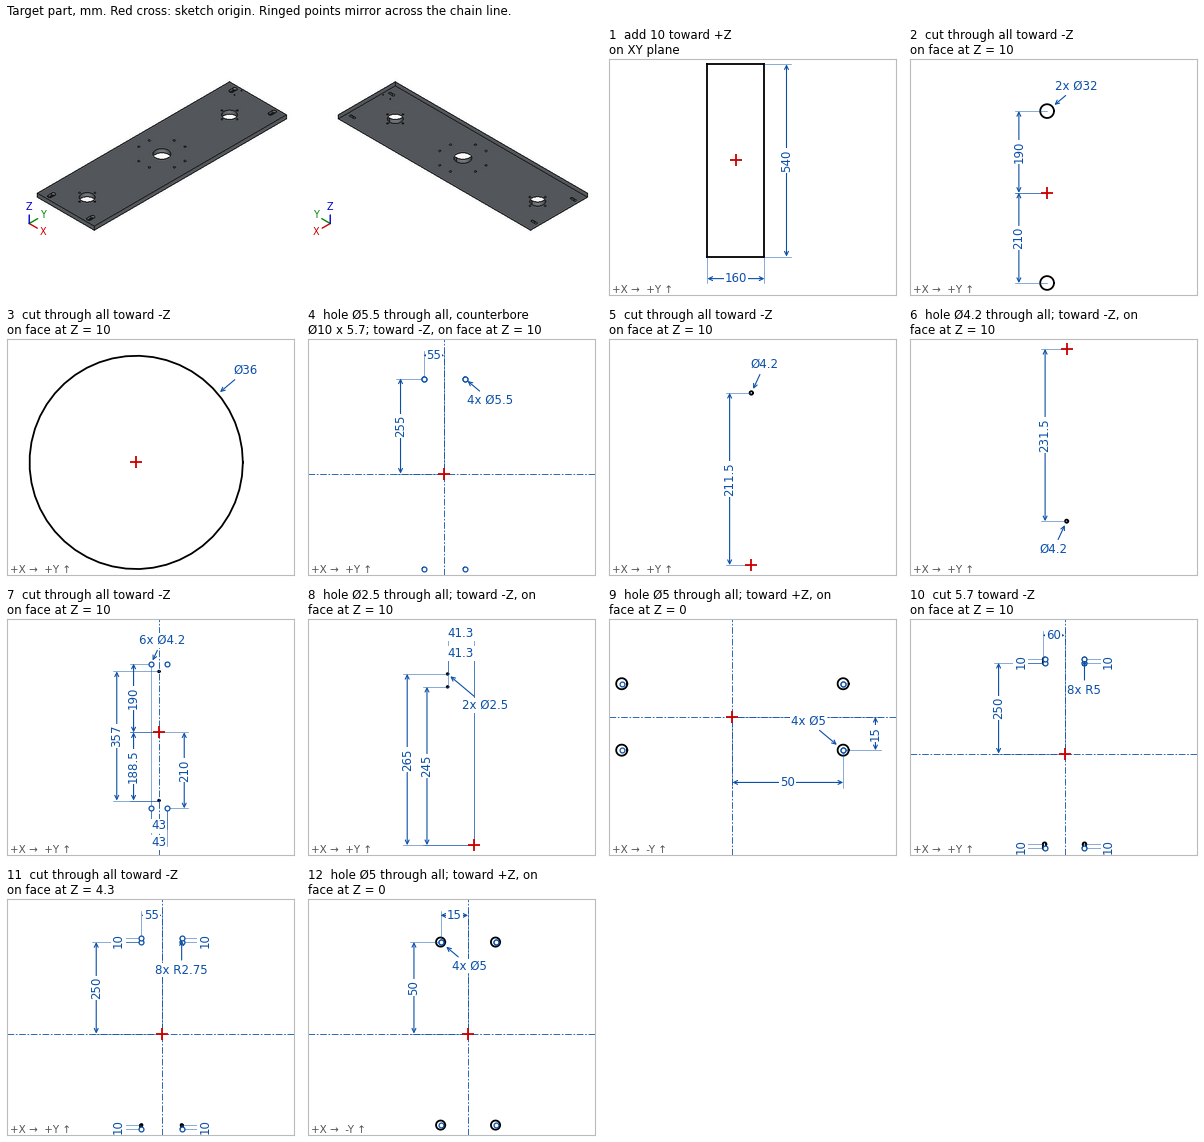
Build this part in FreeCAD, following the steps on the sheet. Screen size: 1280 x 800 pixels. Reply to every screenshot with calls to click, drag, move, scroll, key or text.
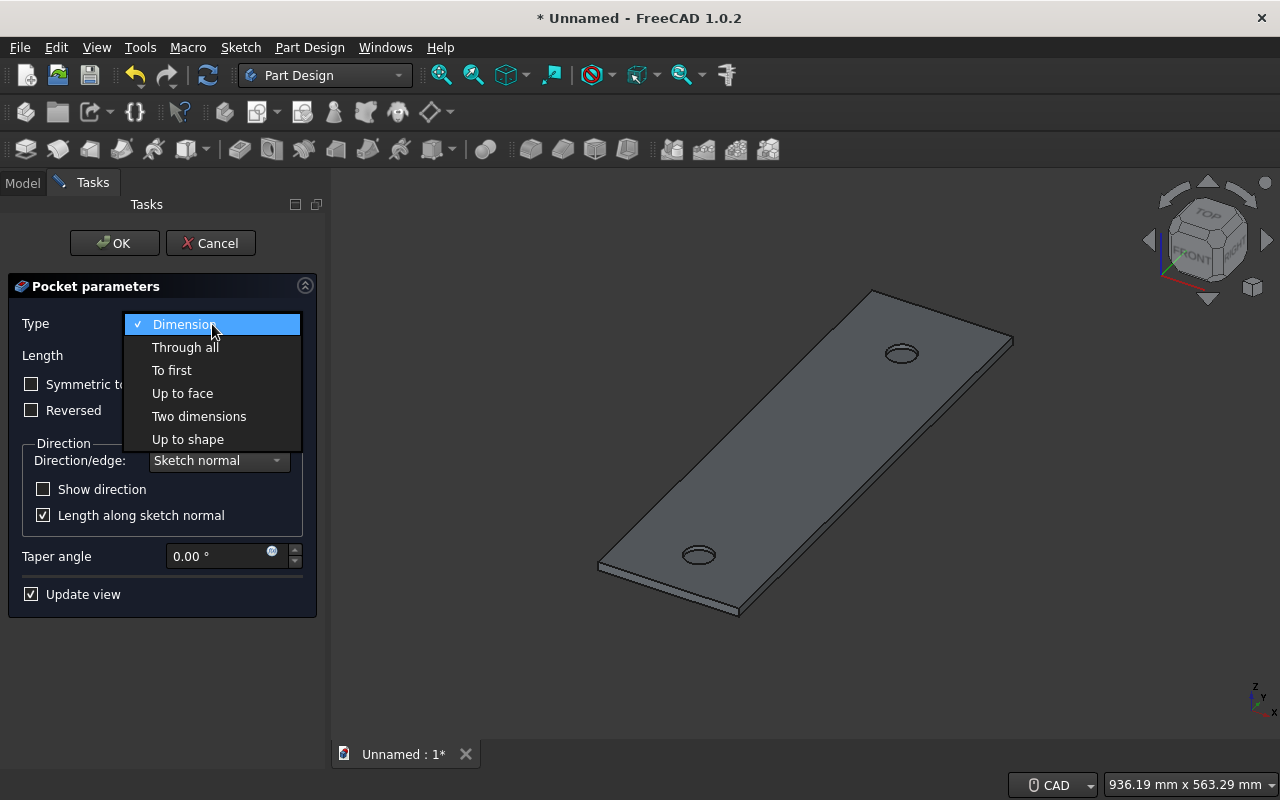
click(212, 348)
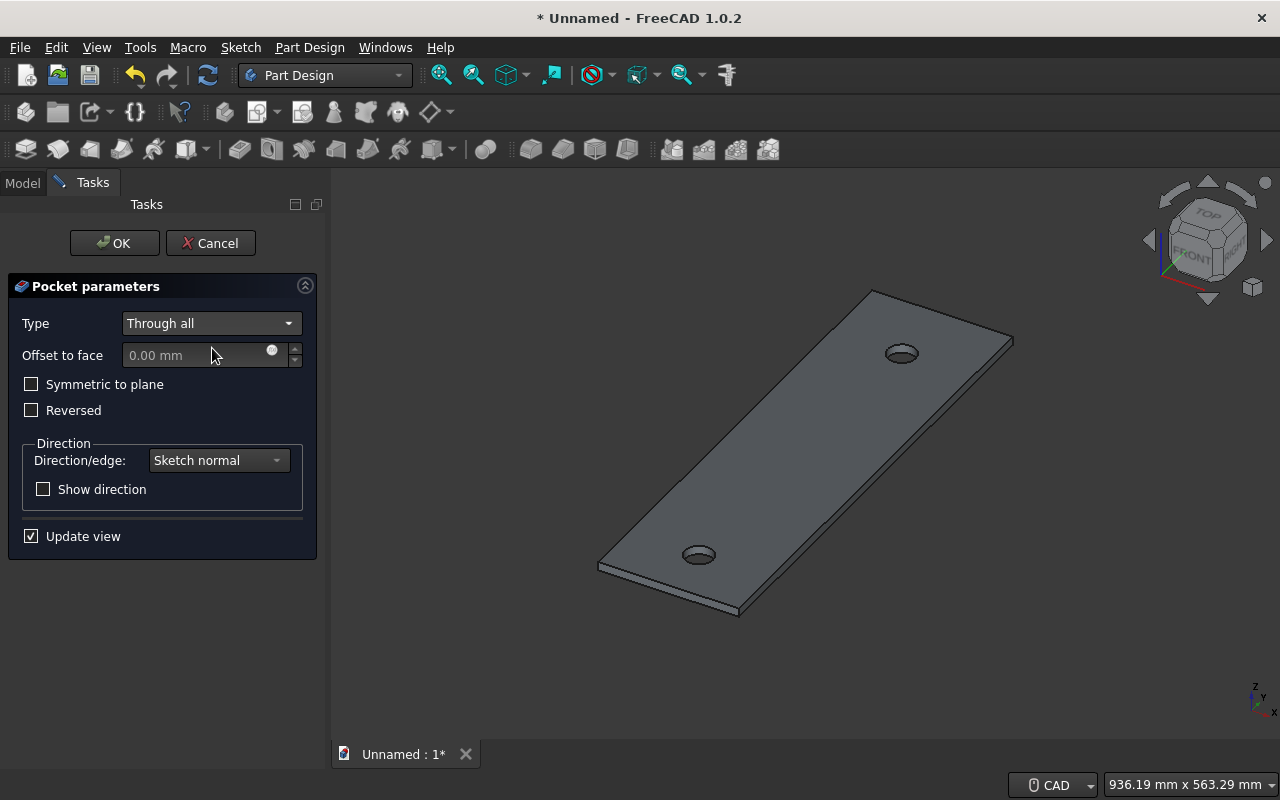
click(115, 243)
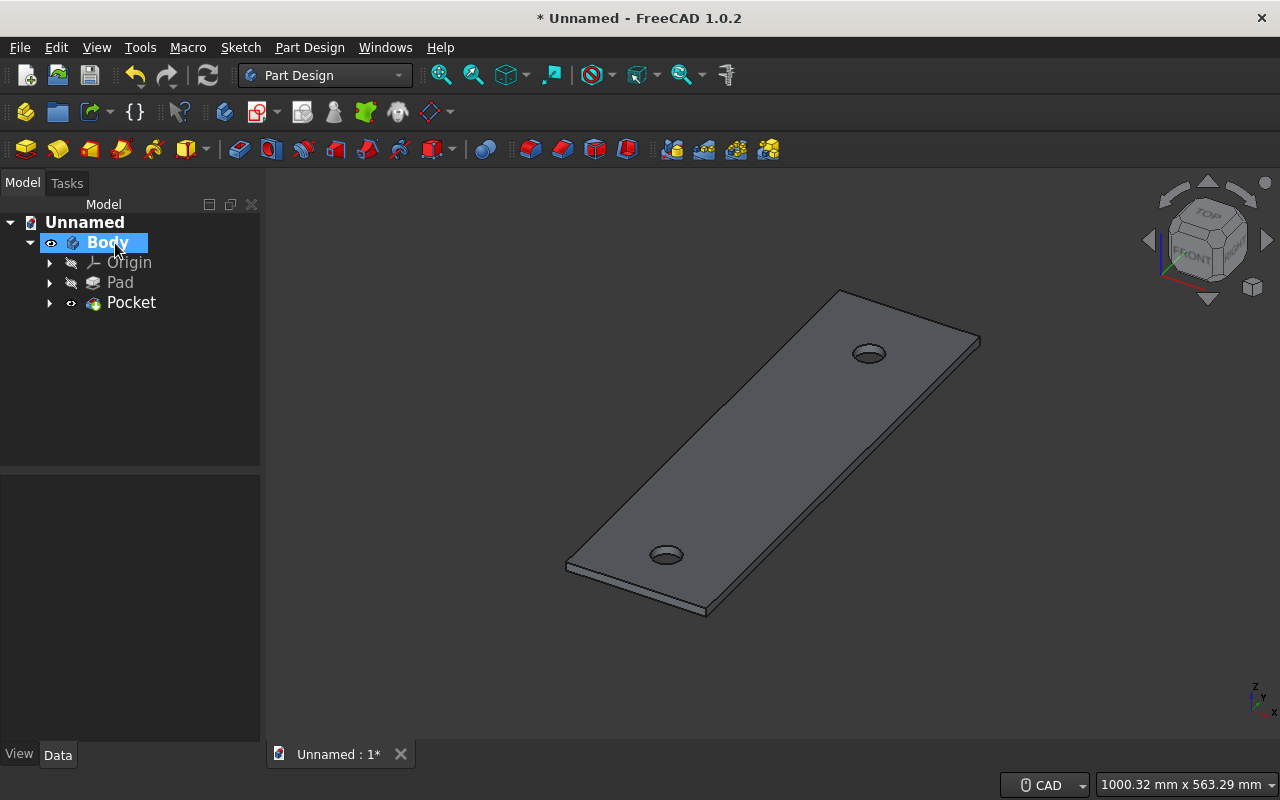
click(812, 410)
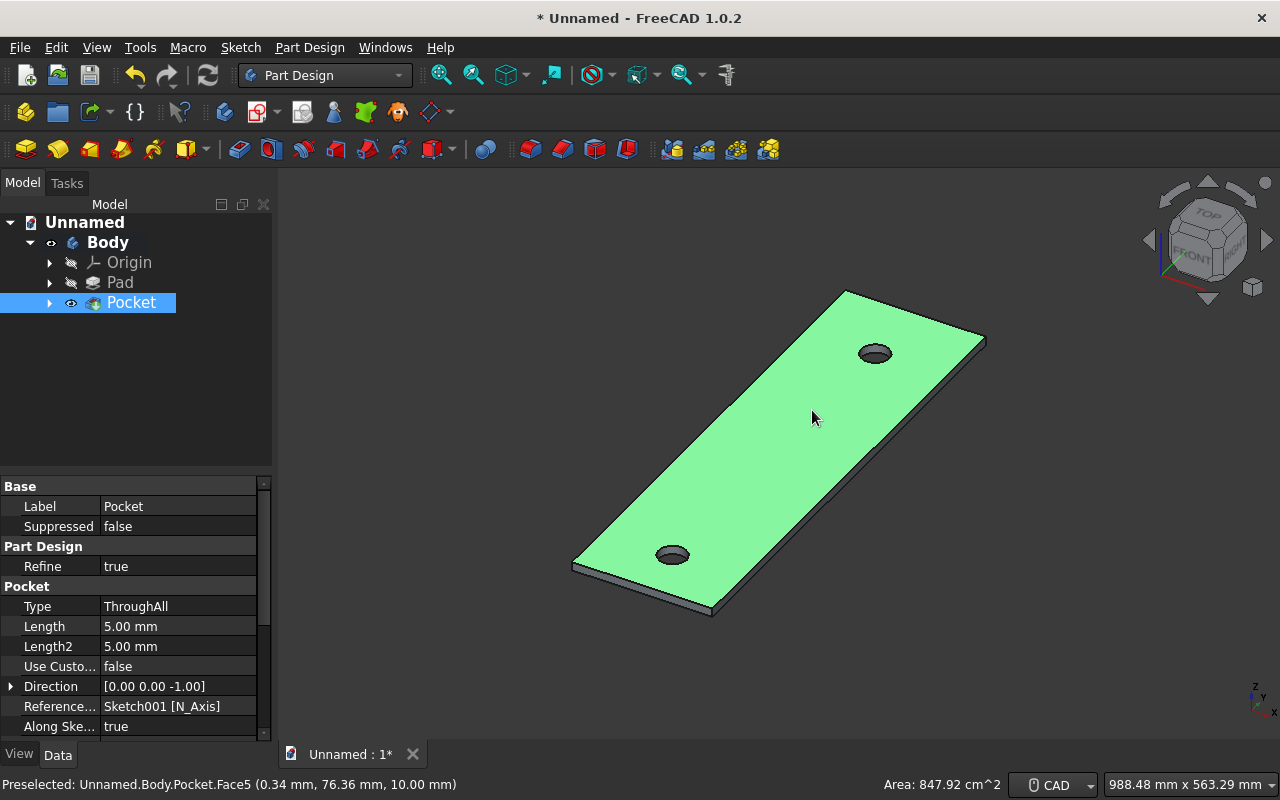
click(258, 112)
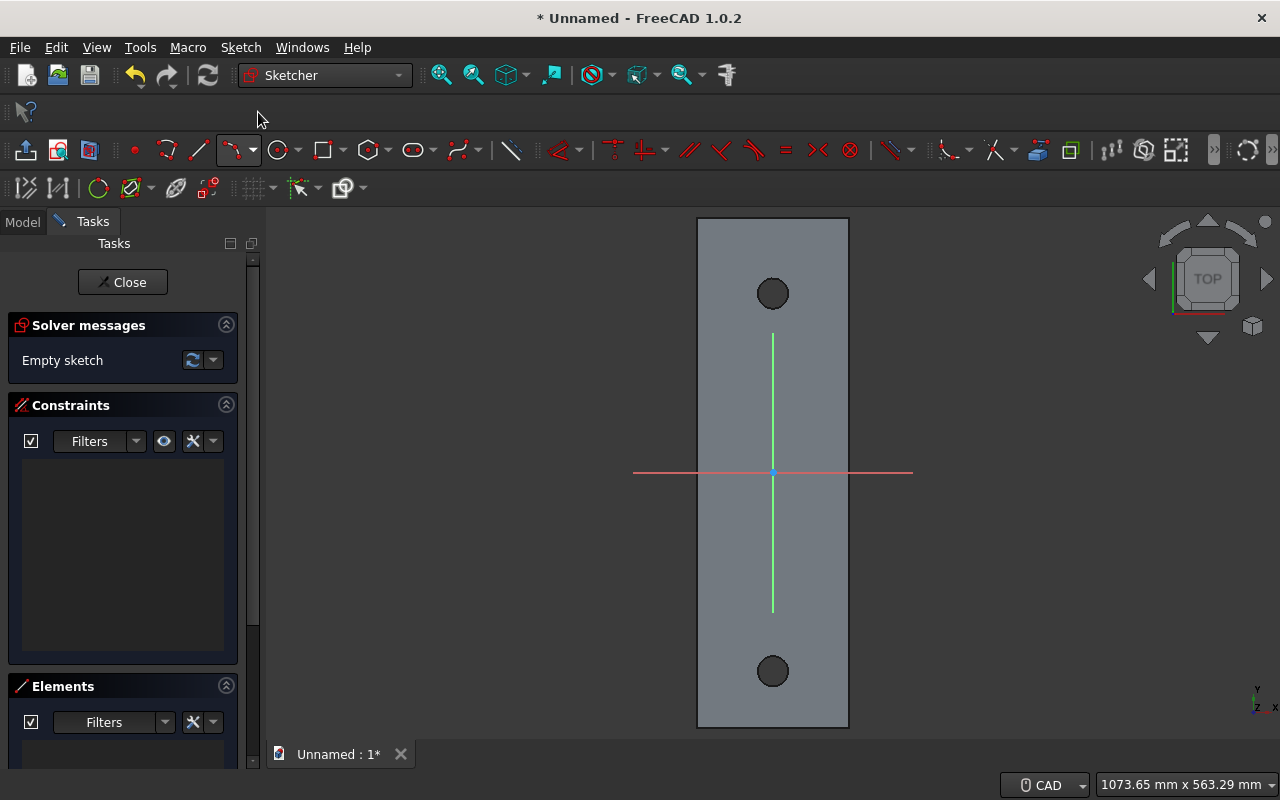
scroll(782, 473, up, 11)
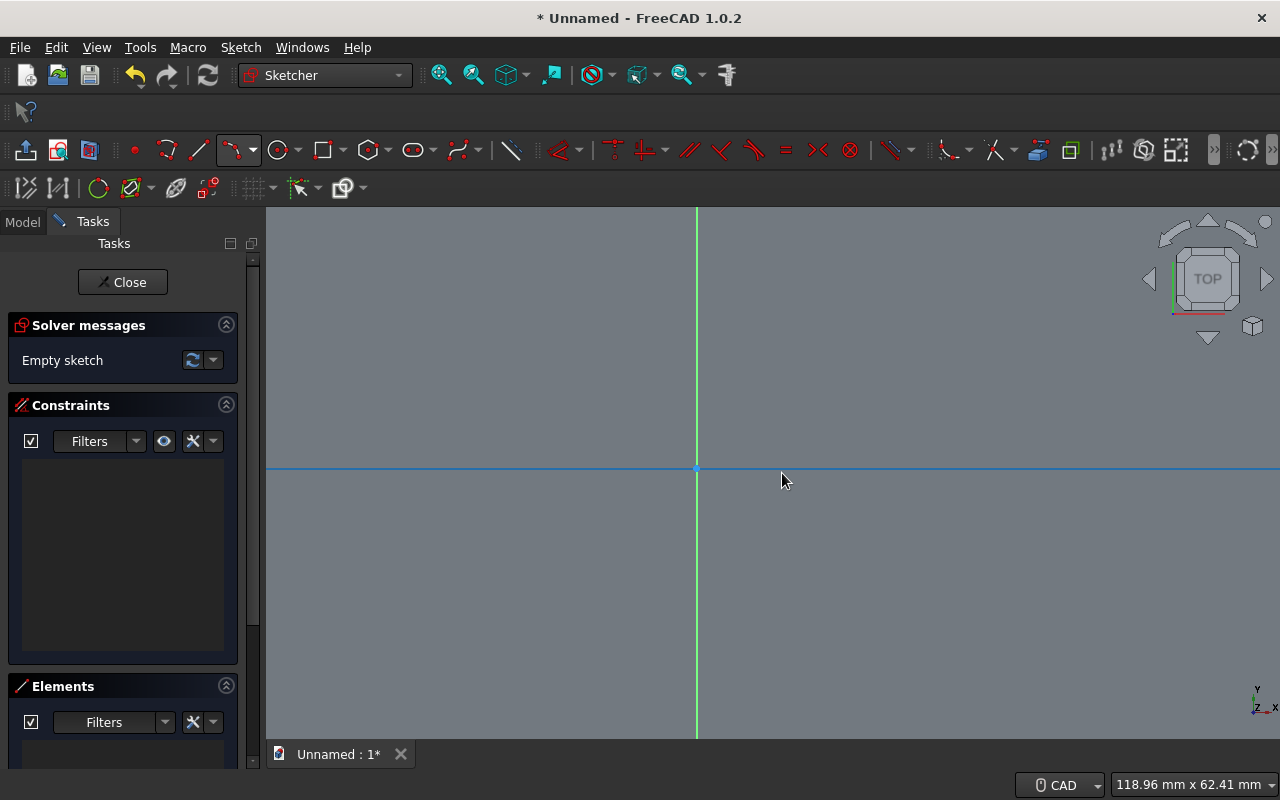
key(g)
key(c)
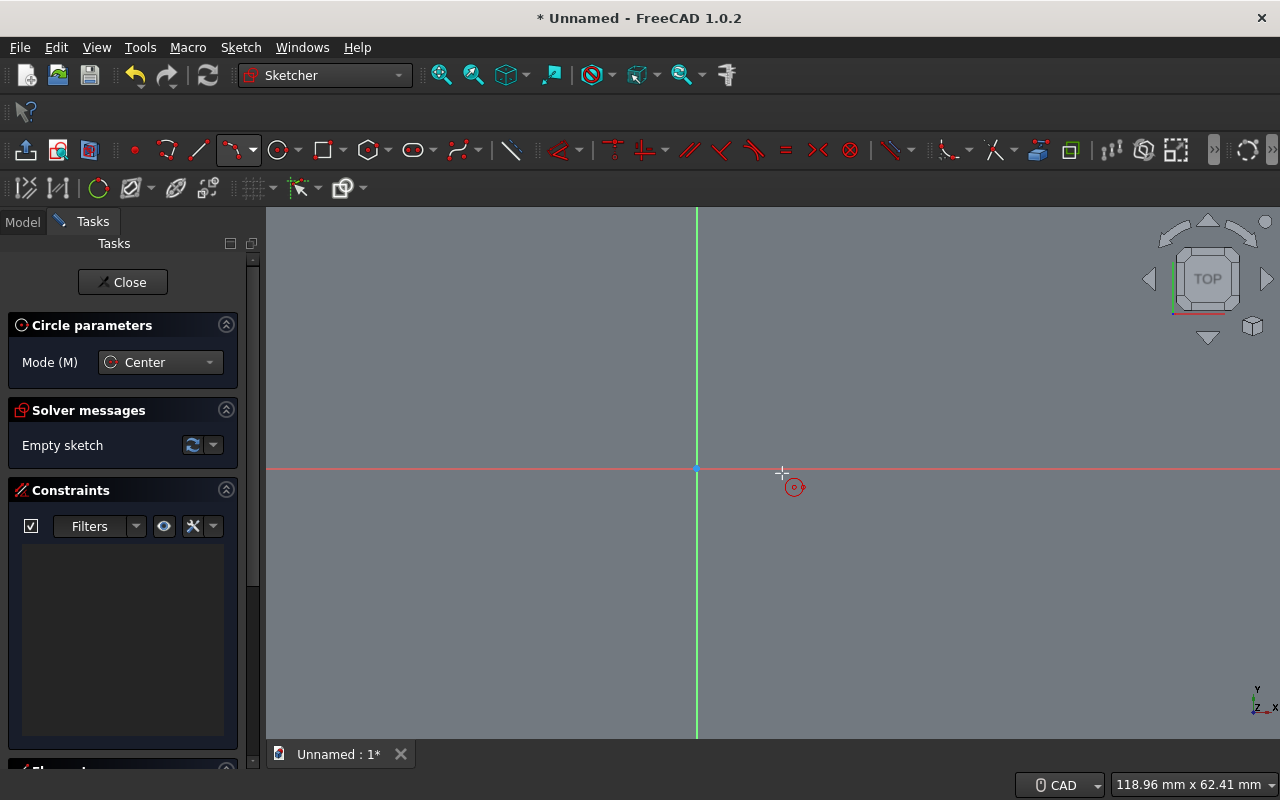
click(697, 469)
move(805, 360)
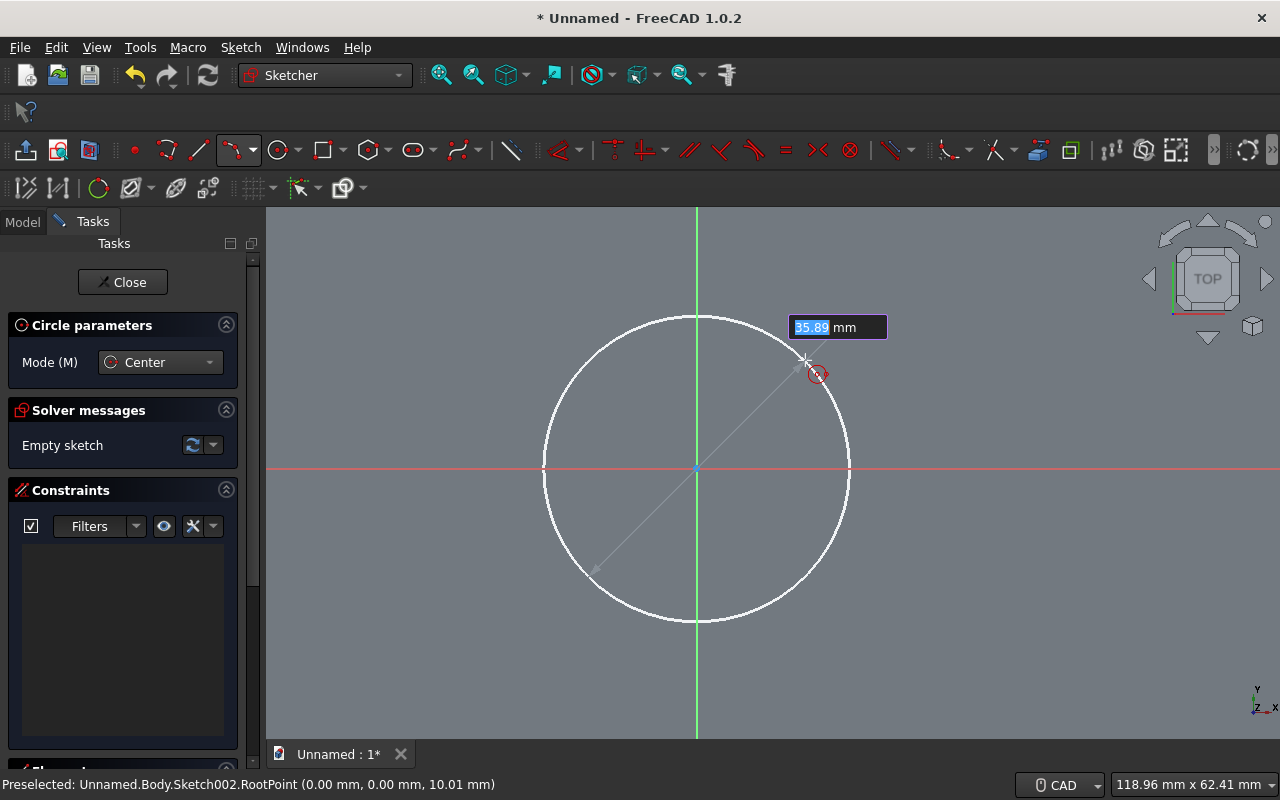
text(36)
key(Return)
key(Escape)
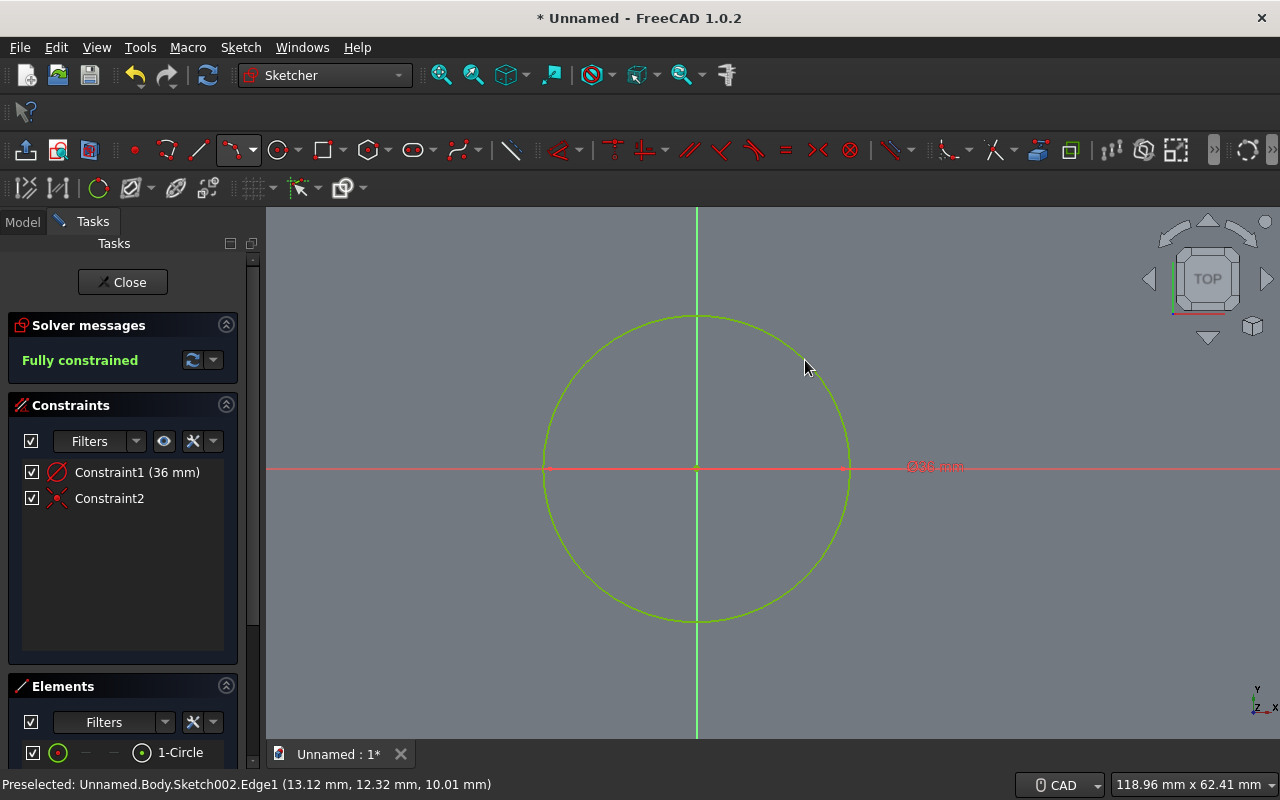
click(123, 282)